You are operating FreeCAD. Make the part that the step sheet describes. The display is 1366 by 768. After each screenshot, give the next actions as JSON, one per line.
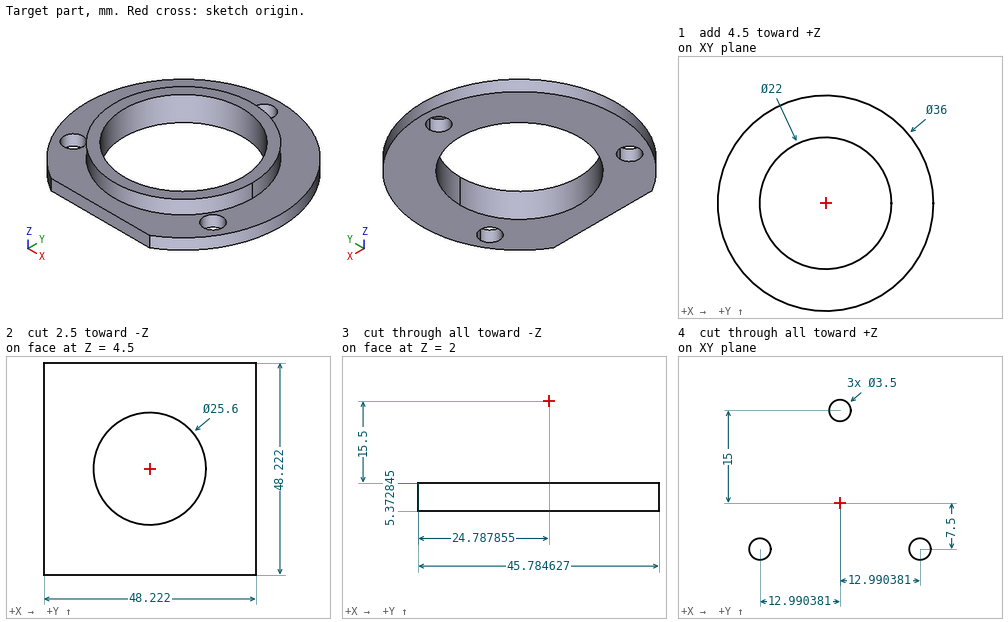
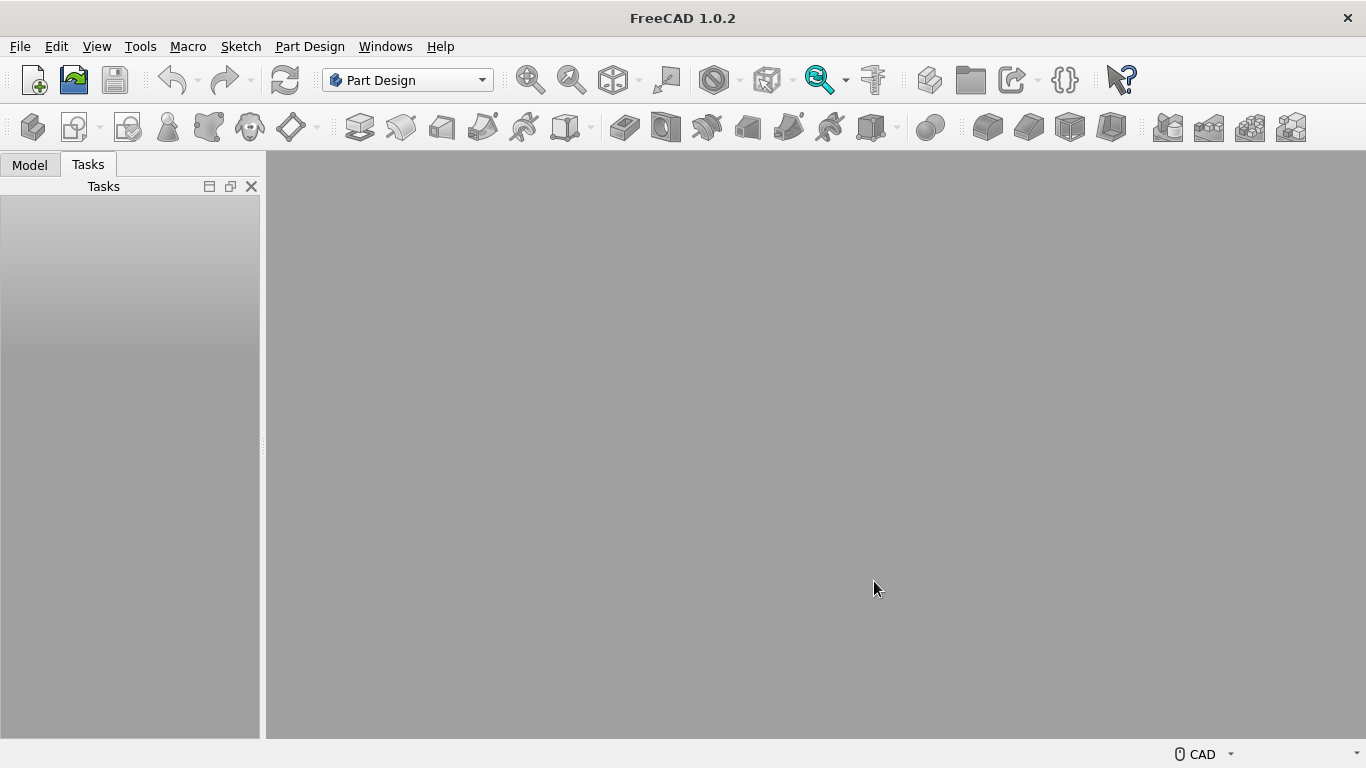
{"action": "left_click", "coordinate": [33, 80]}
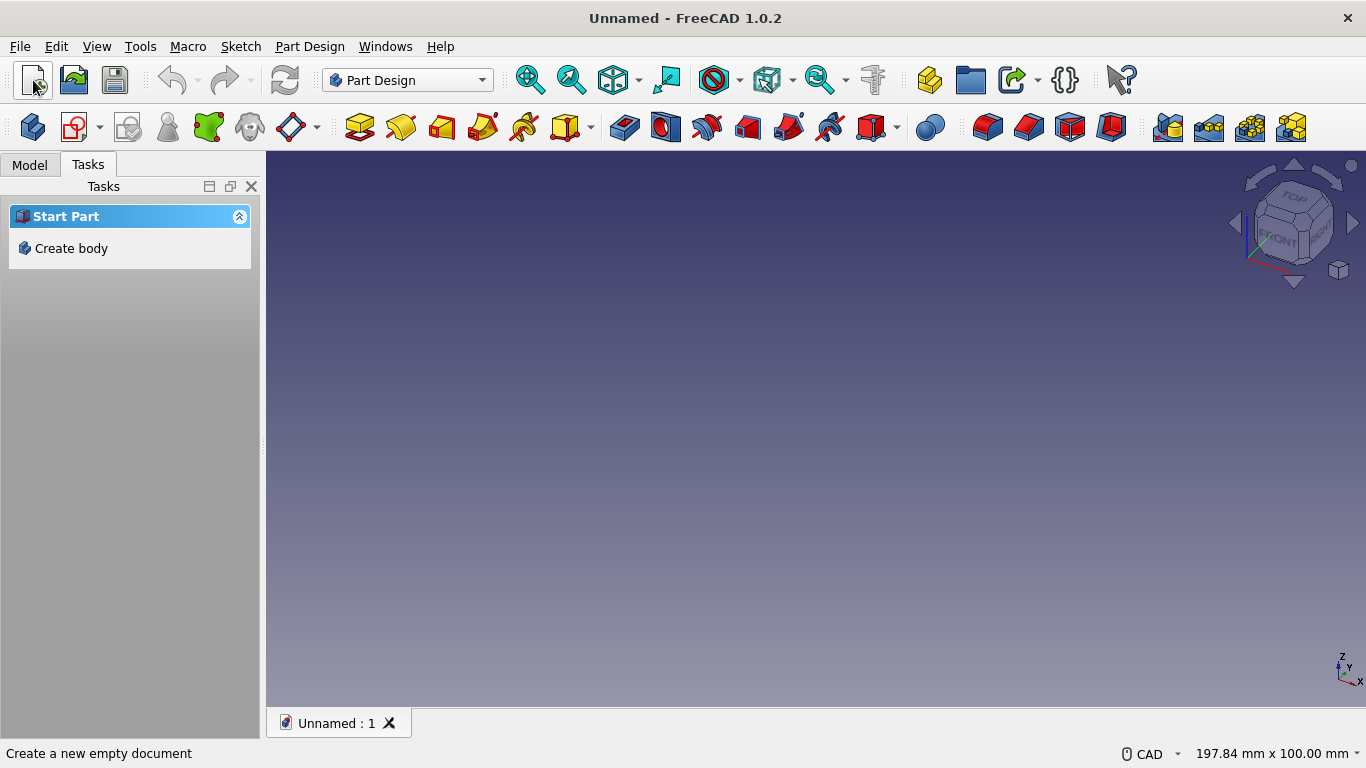
{"action": "left_click", "coordinate": [74, 128]}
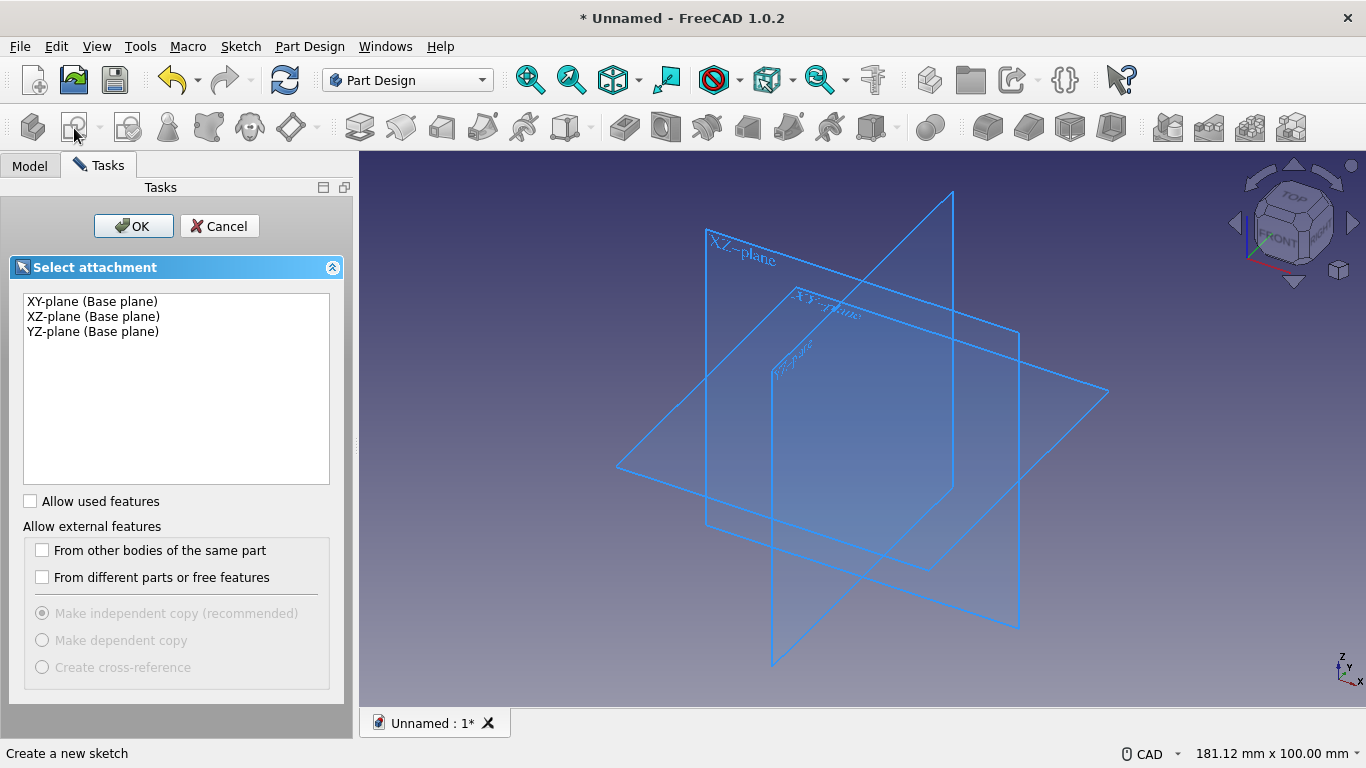
{"action": "left_click", "coordinate": [84, 302]}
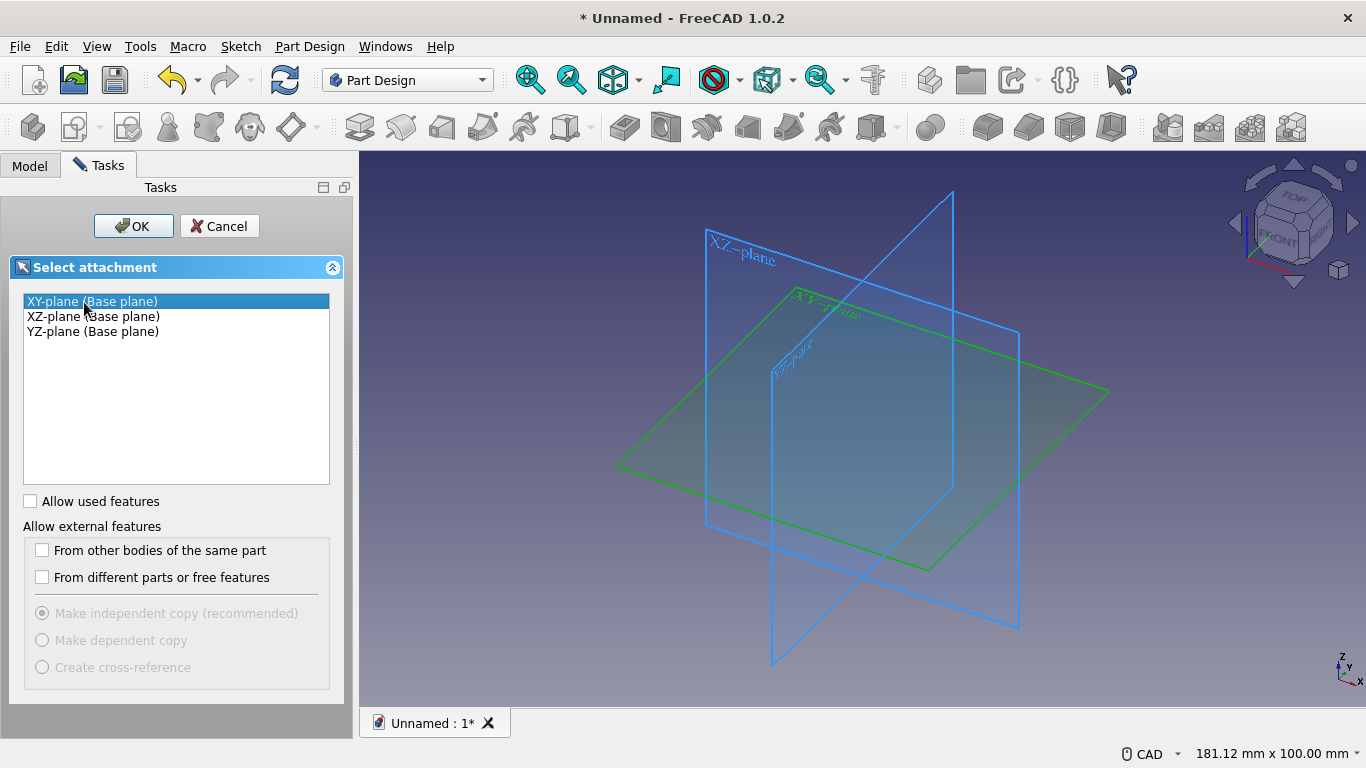
{"action": "left_click", "coordinate": [134, 226]}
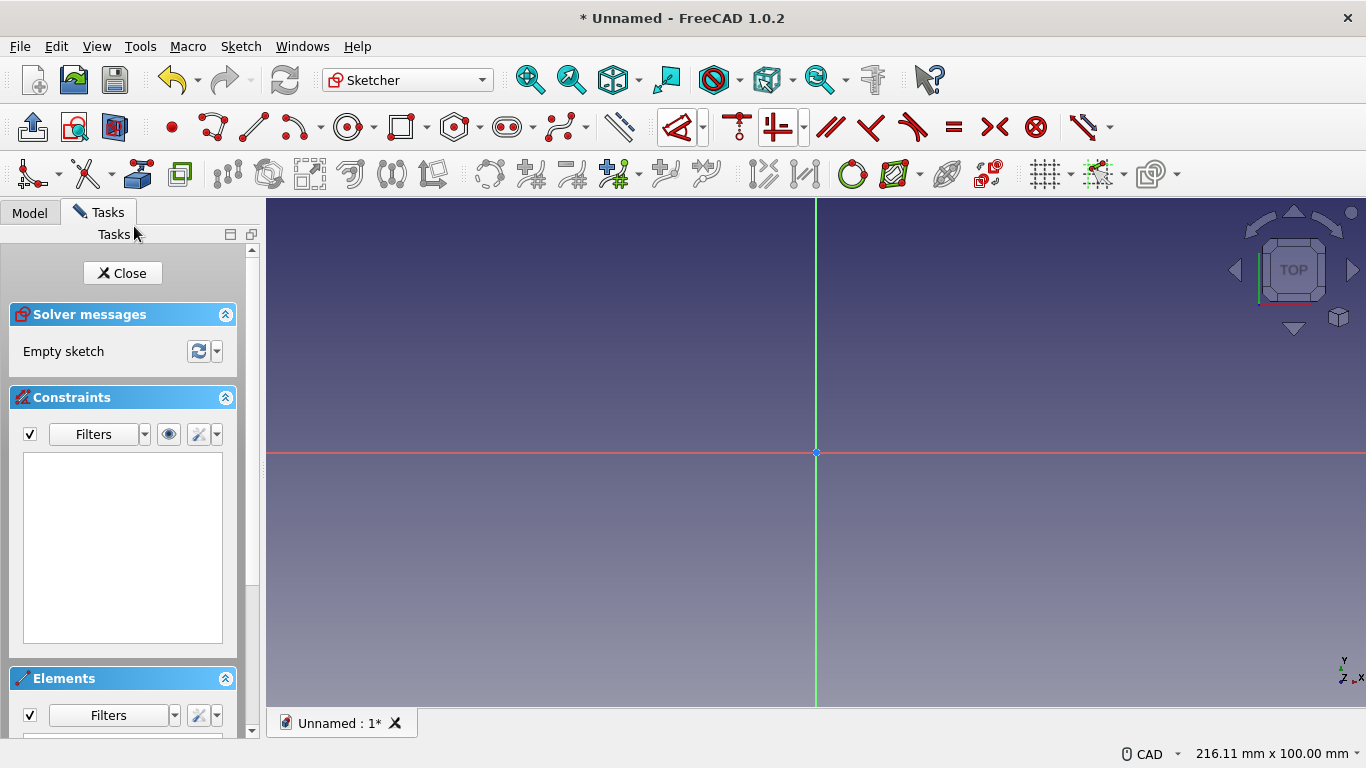
{"action": "scroll", "coordinate": [899, 452], "scroll_direction": "up", "scroll_amount": 3}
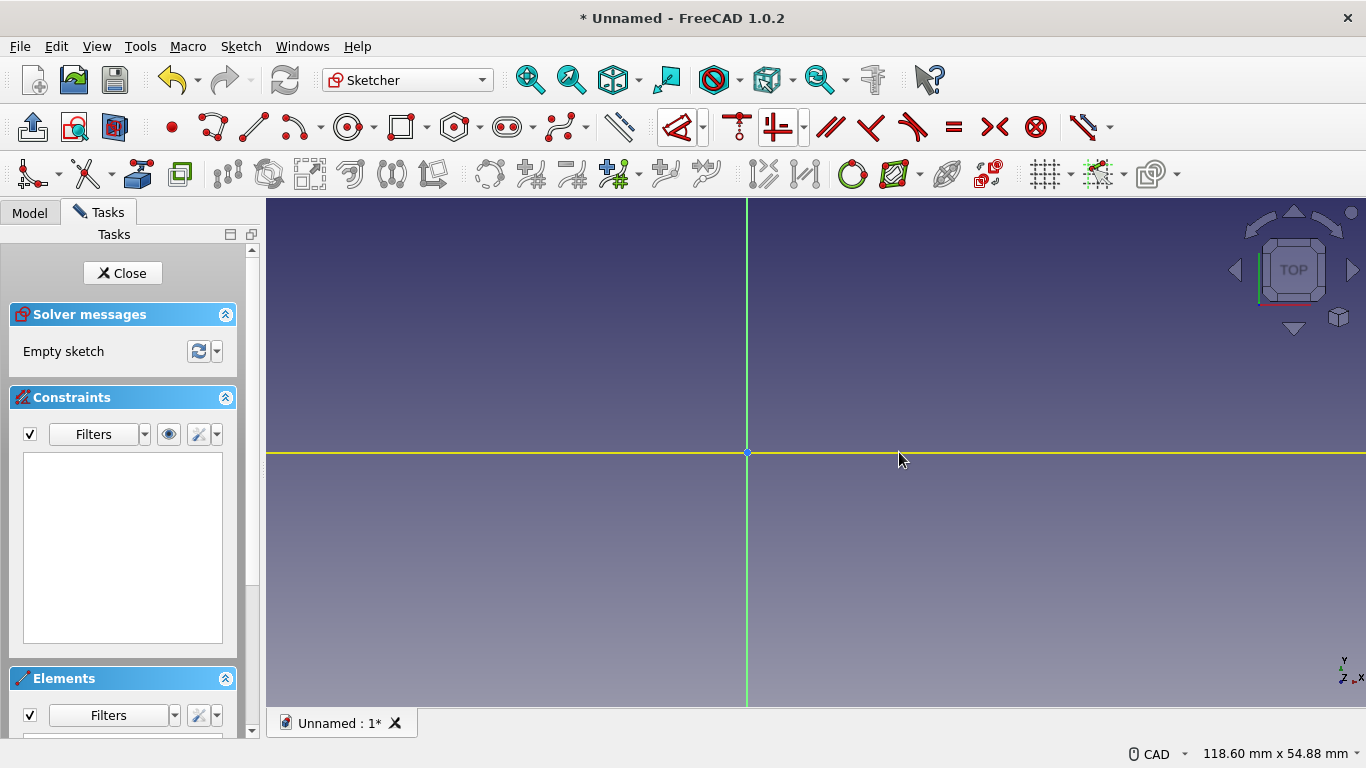
{"action": "key", "text": "g c"}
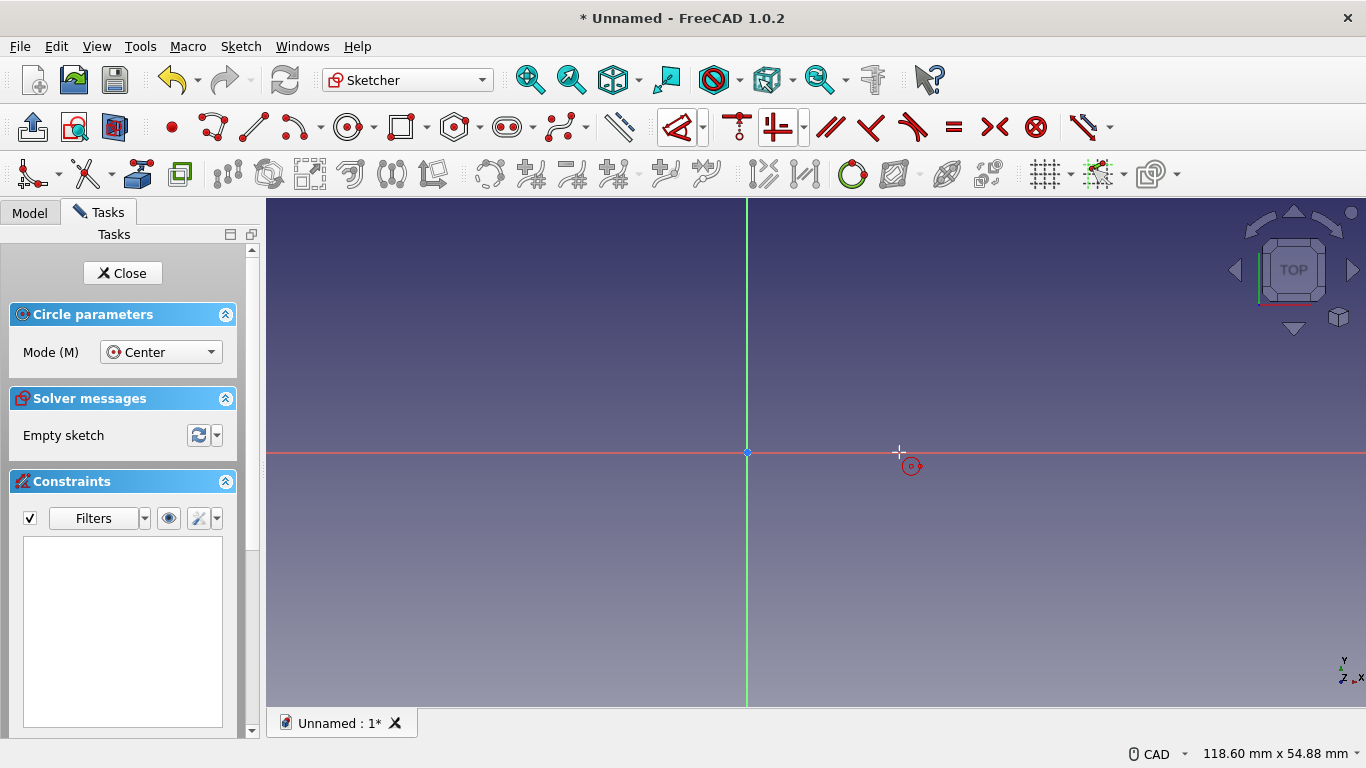
{"action": "left_click", "coordinate": [747, 452]}
{"action": "left_click", "coordinate": [865, 334]}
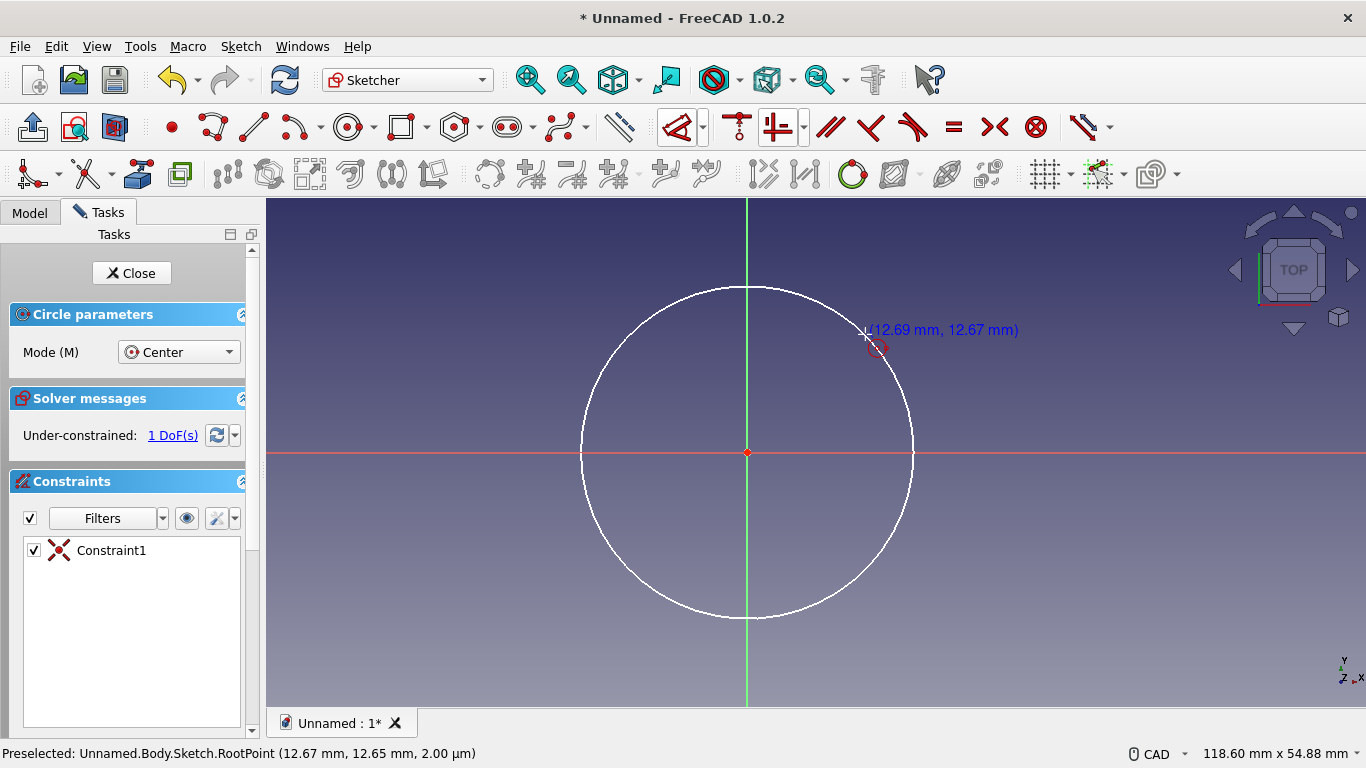
{"action": "left_click", "coordinate": [747, 452]}
{"action": "left_click", "coordinate": [819, 380]}
{"action": "key", "text": "Escape"}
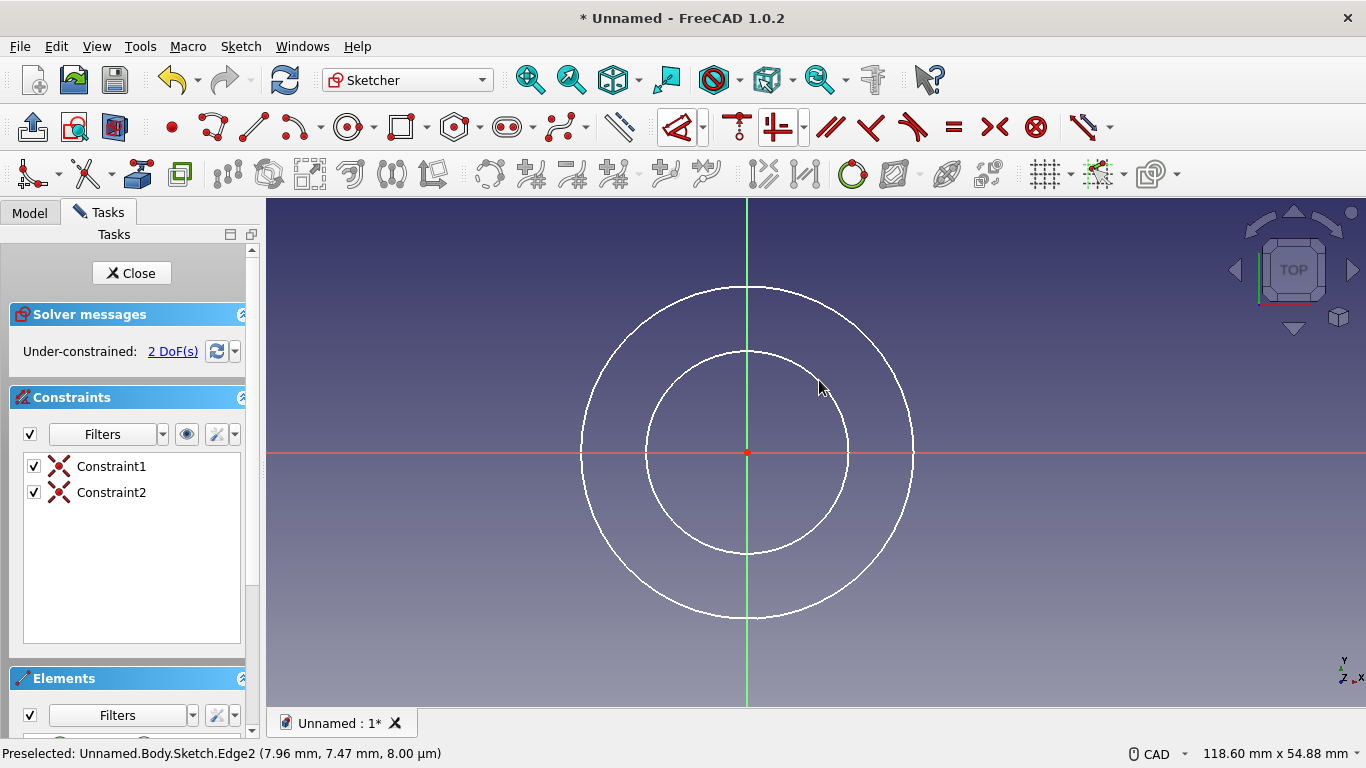
{"action": "left_click", "coordinate": [676, 128]}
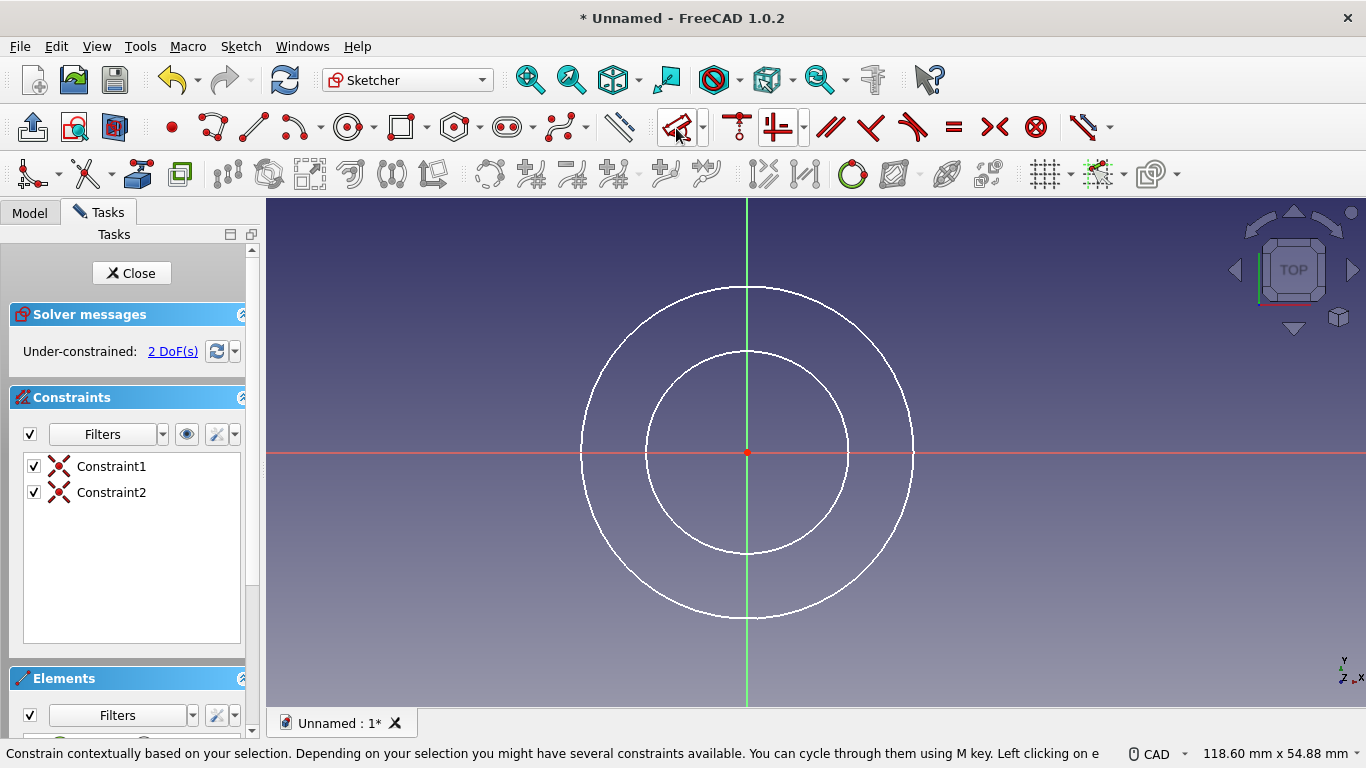
{"action": "left_click", "coordinate": [865, 335]}
{"action": "left_click", "coordinate": [888, 312]}